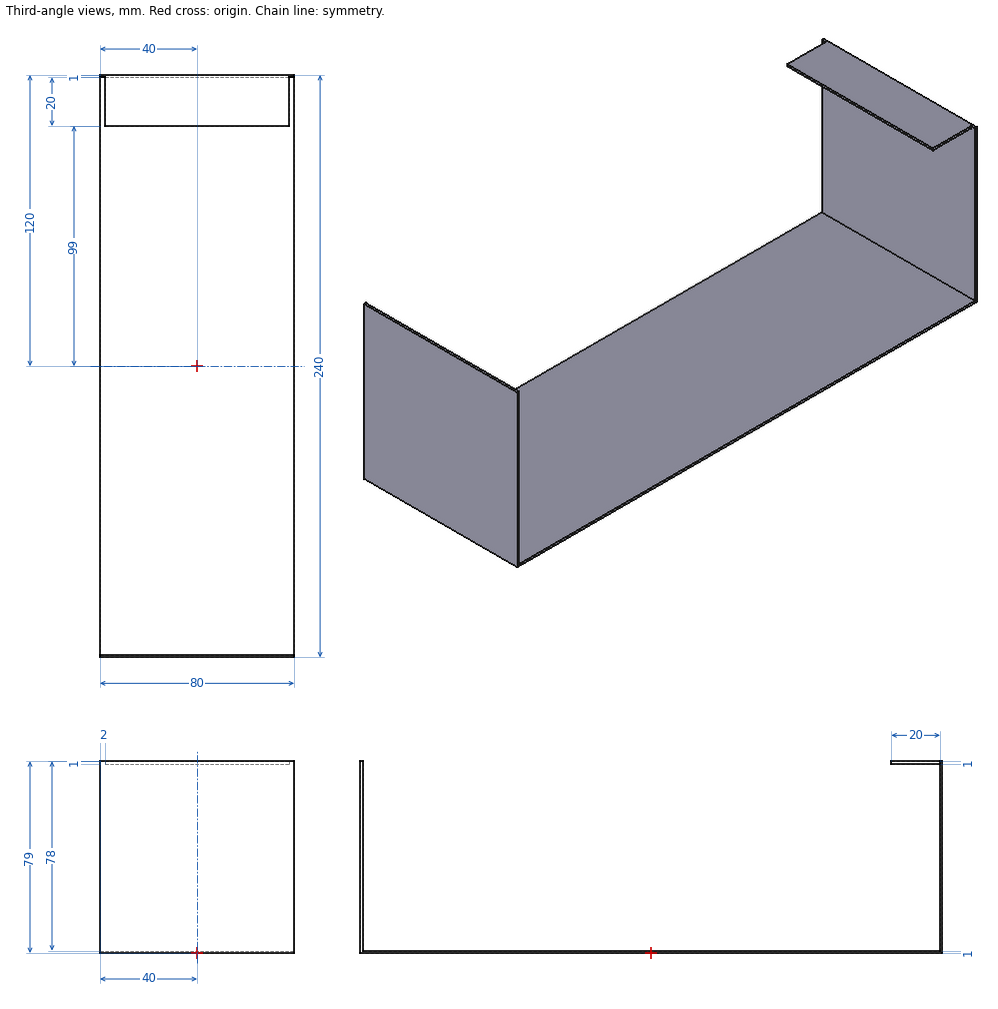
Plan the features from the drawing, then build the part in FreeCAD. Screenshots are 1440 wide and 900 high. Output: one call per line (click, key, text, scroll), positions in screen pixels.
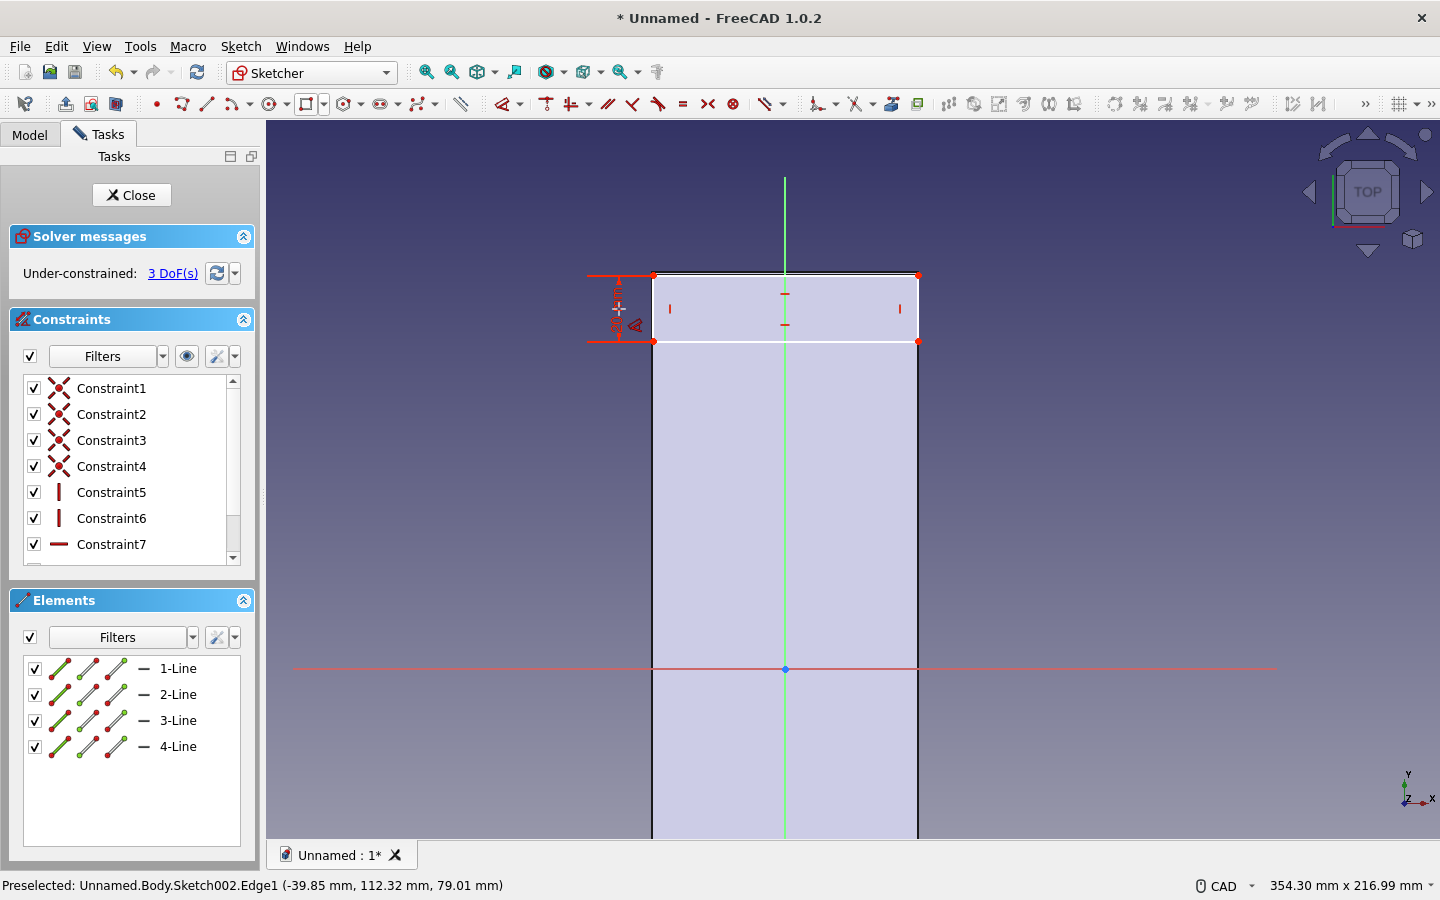
click(732, 342)
click(725, 308)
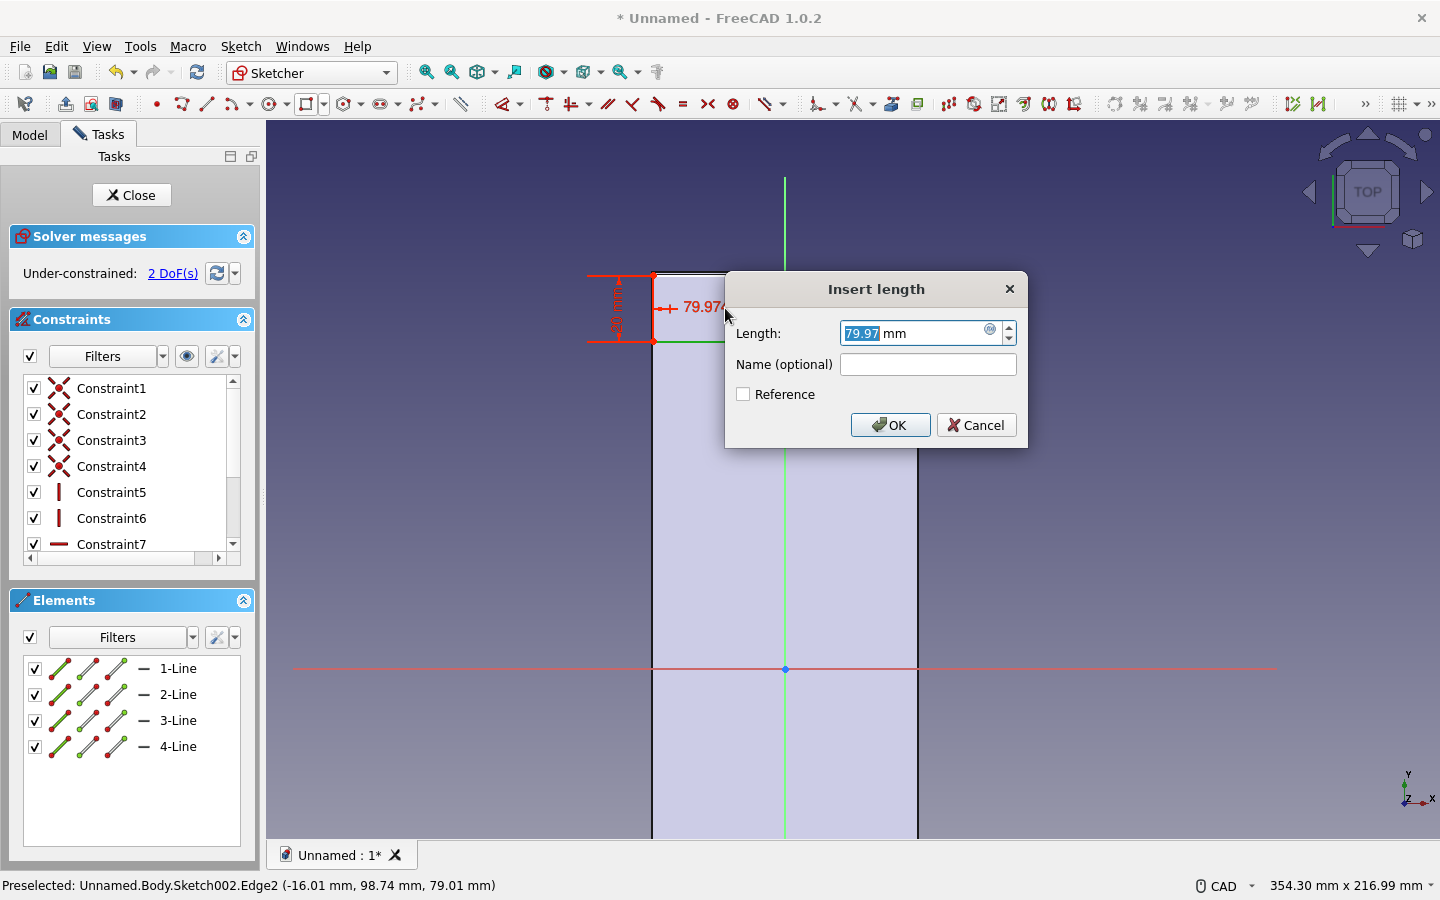
text(80)
key(Return)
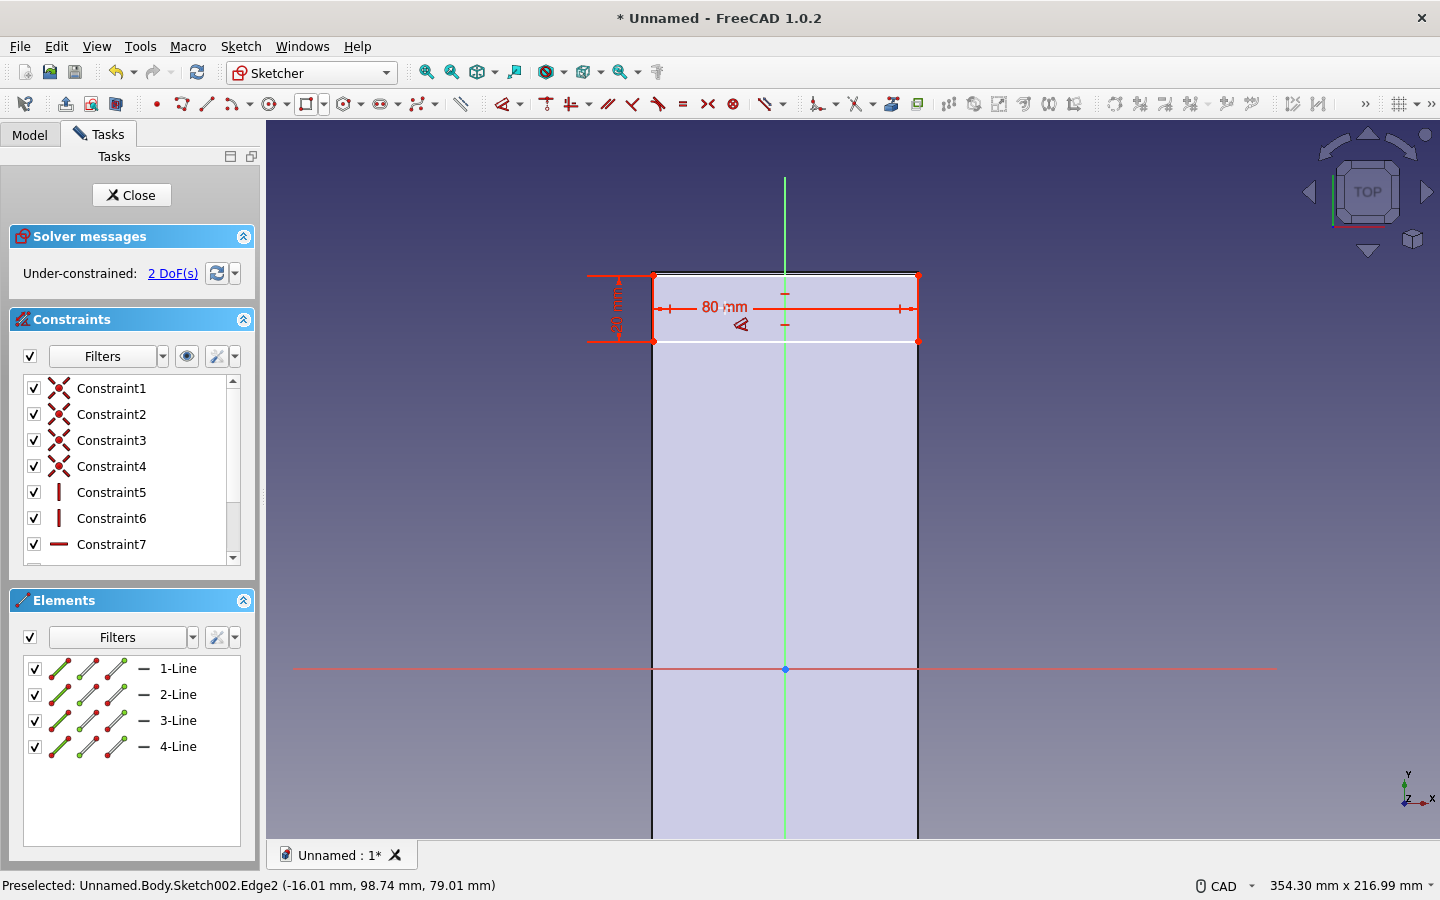
click(653, 276)
click(719, 703)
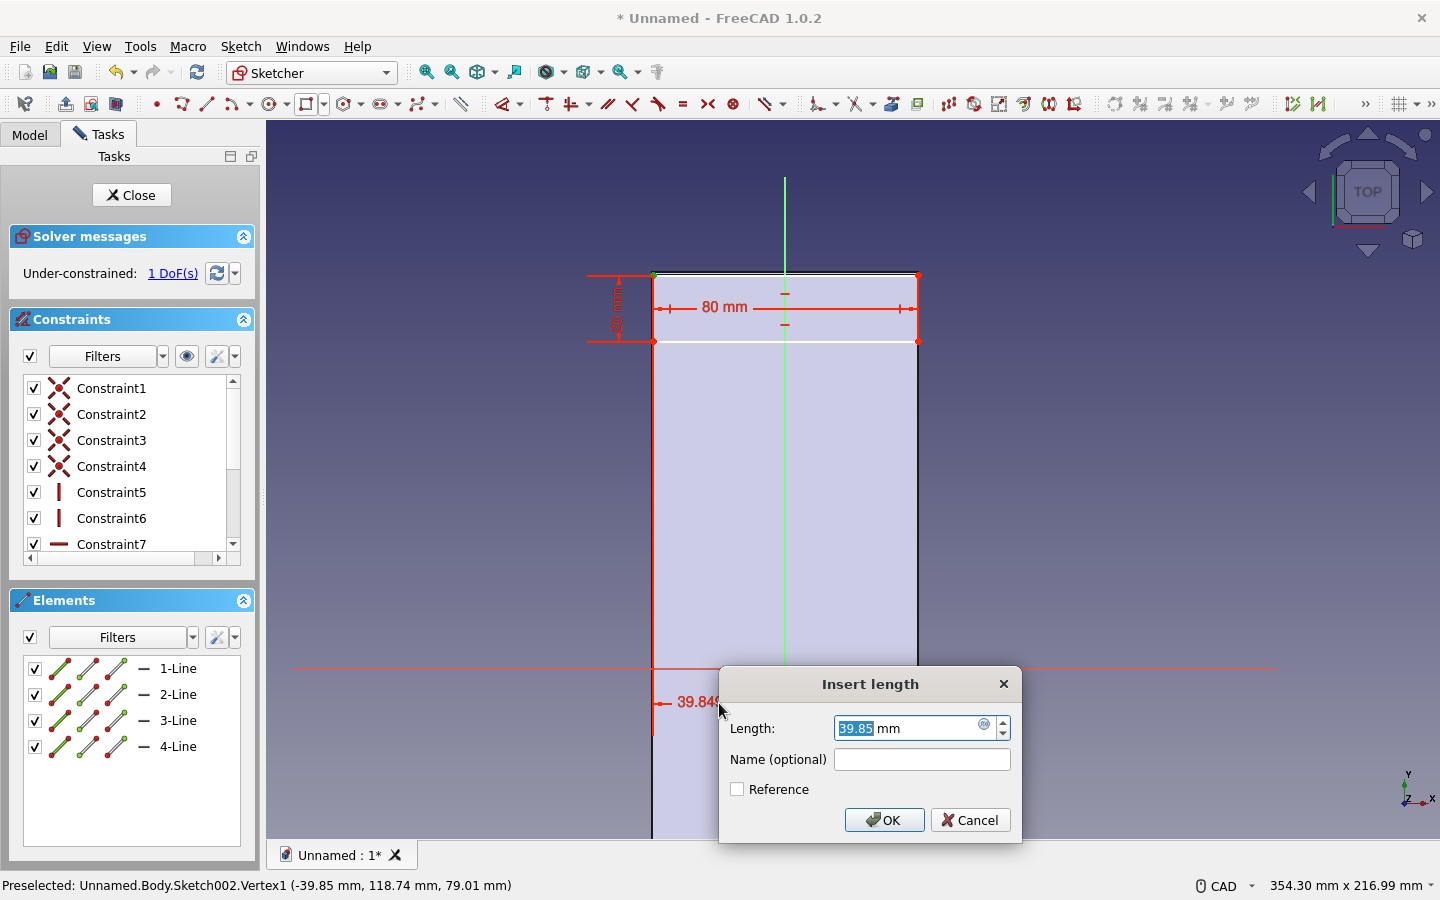
text(40)
key(Return)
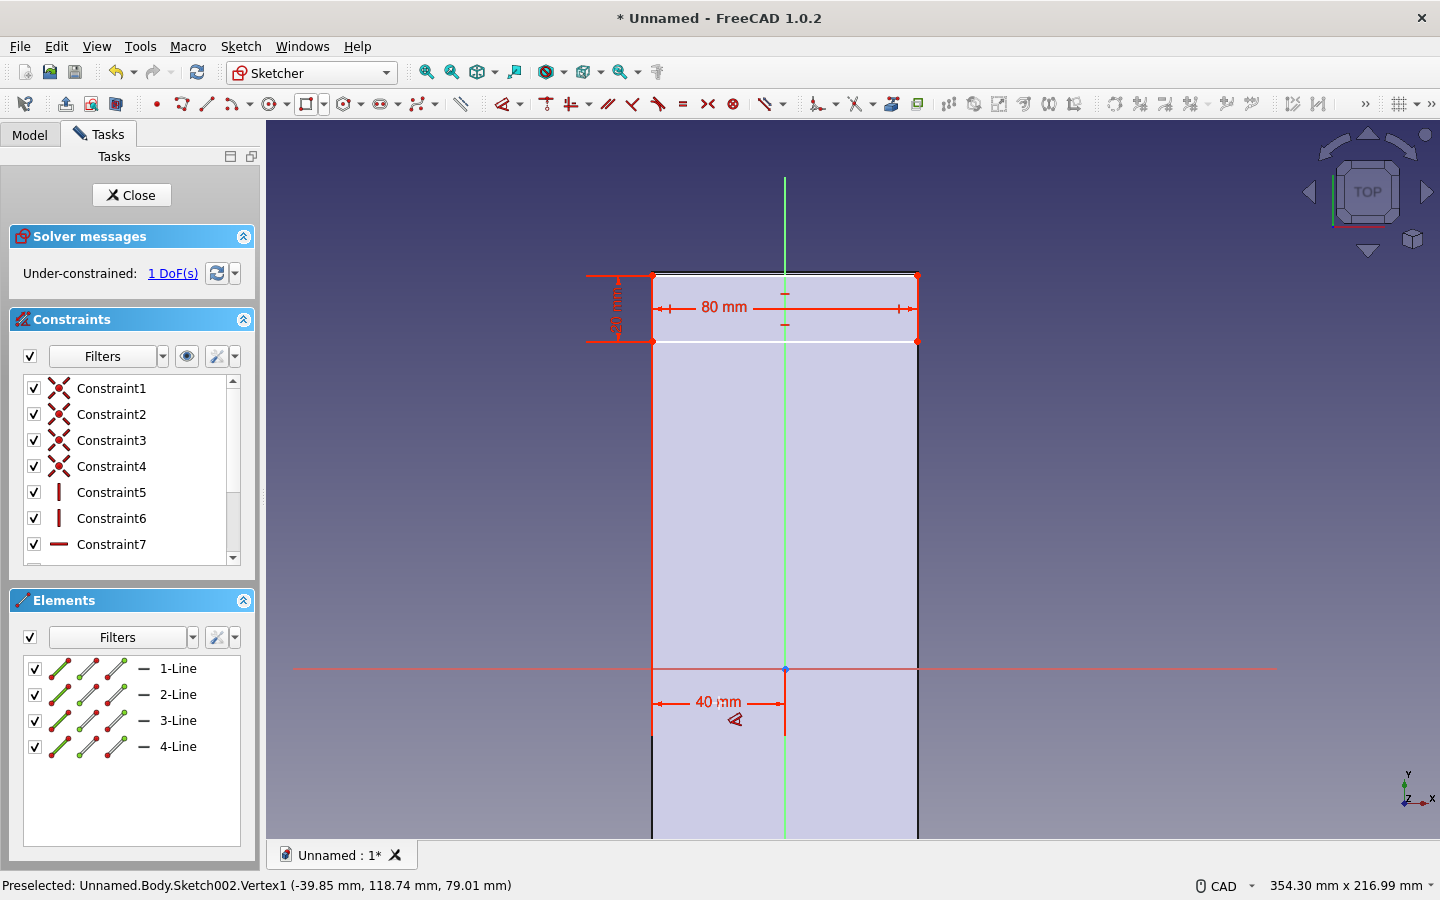
click(653, 342)
click(619, 506)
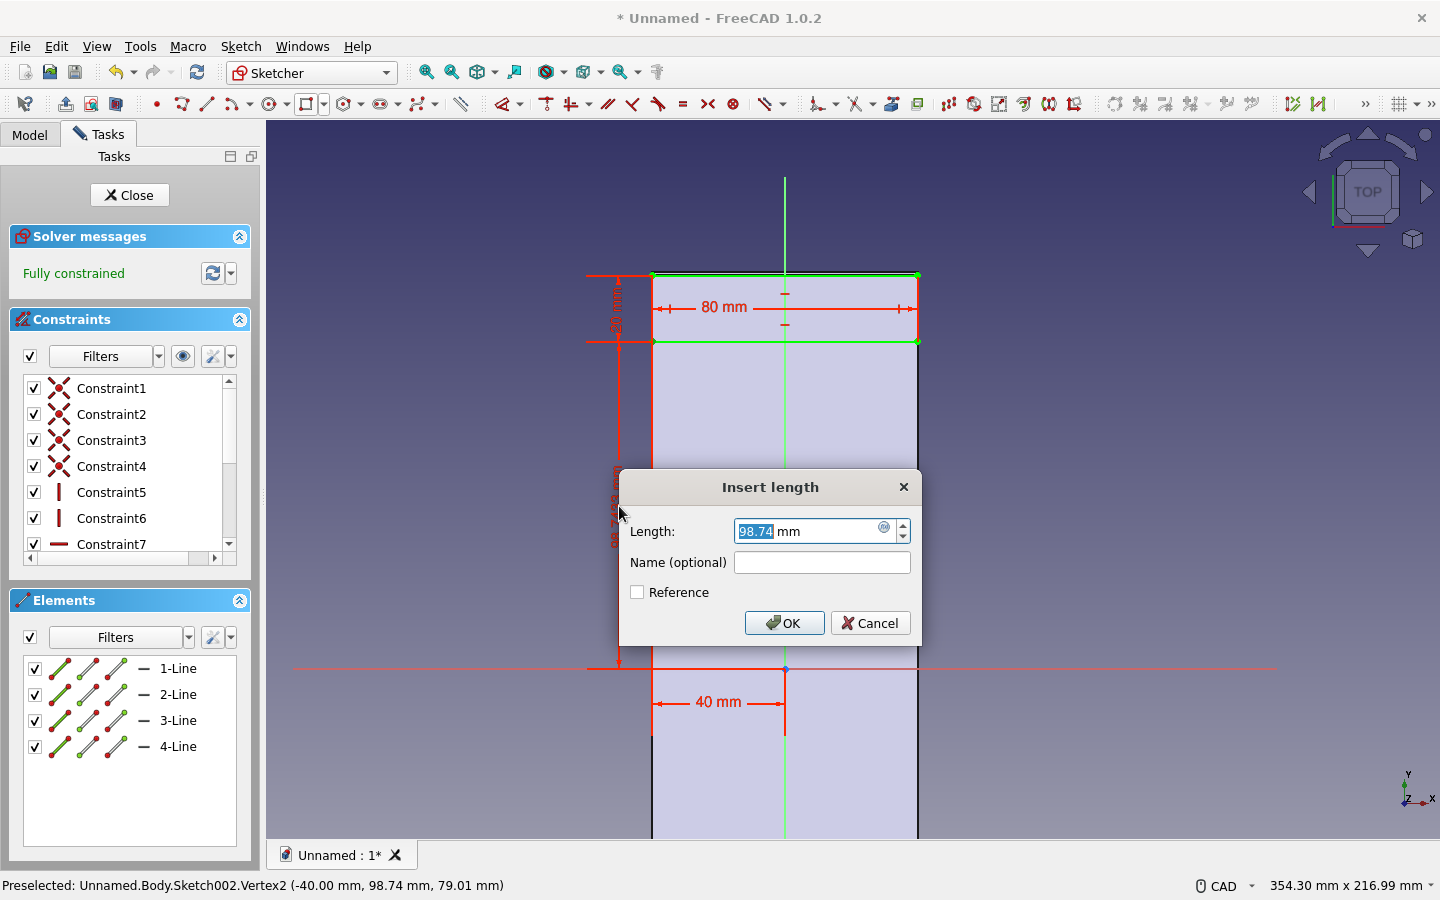
text(99)
key(Return)
key(Escape)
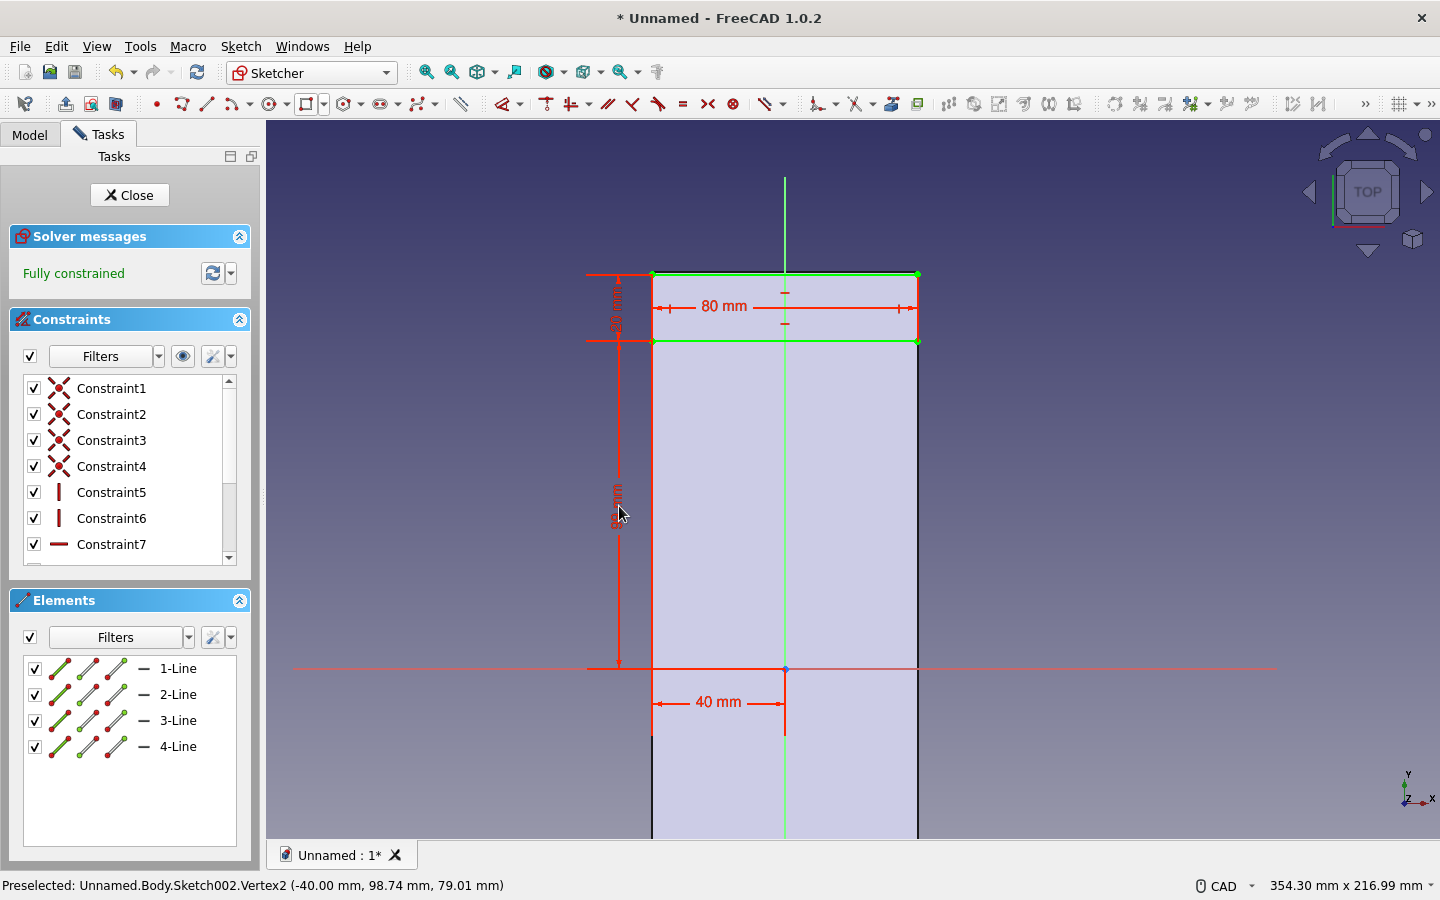
click(130, 195)